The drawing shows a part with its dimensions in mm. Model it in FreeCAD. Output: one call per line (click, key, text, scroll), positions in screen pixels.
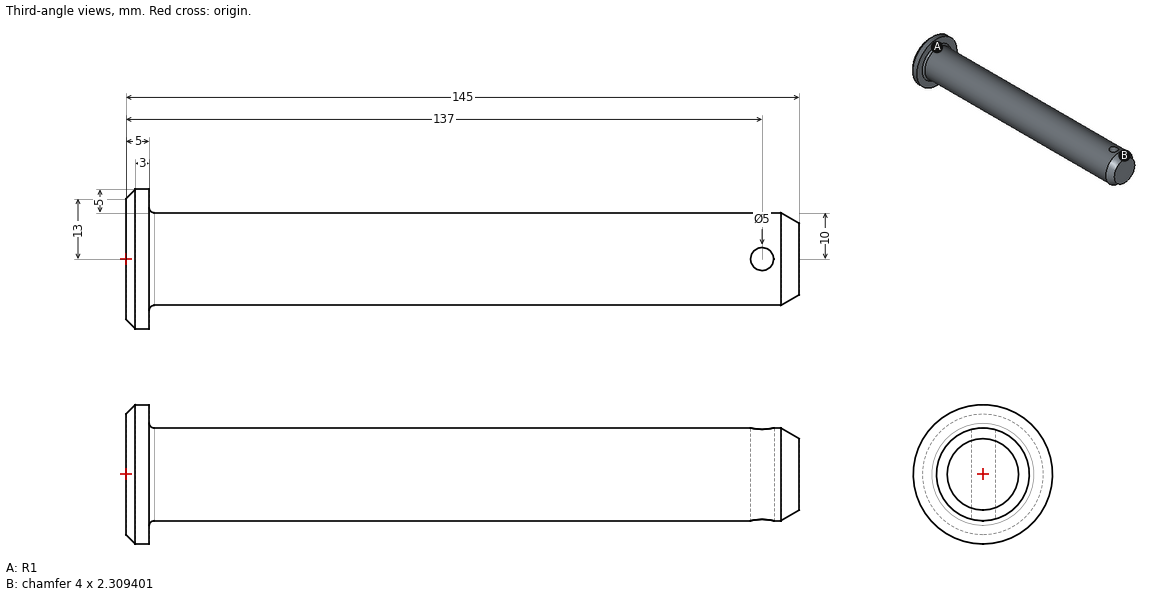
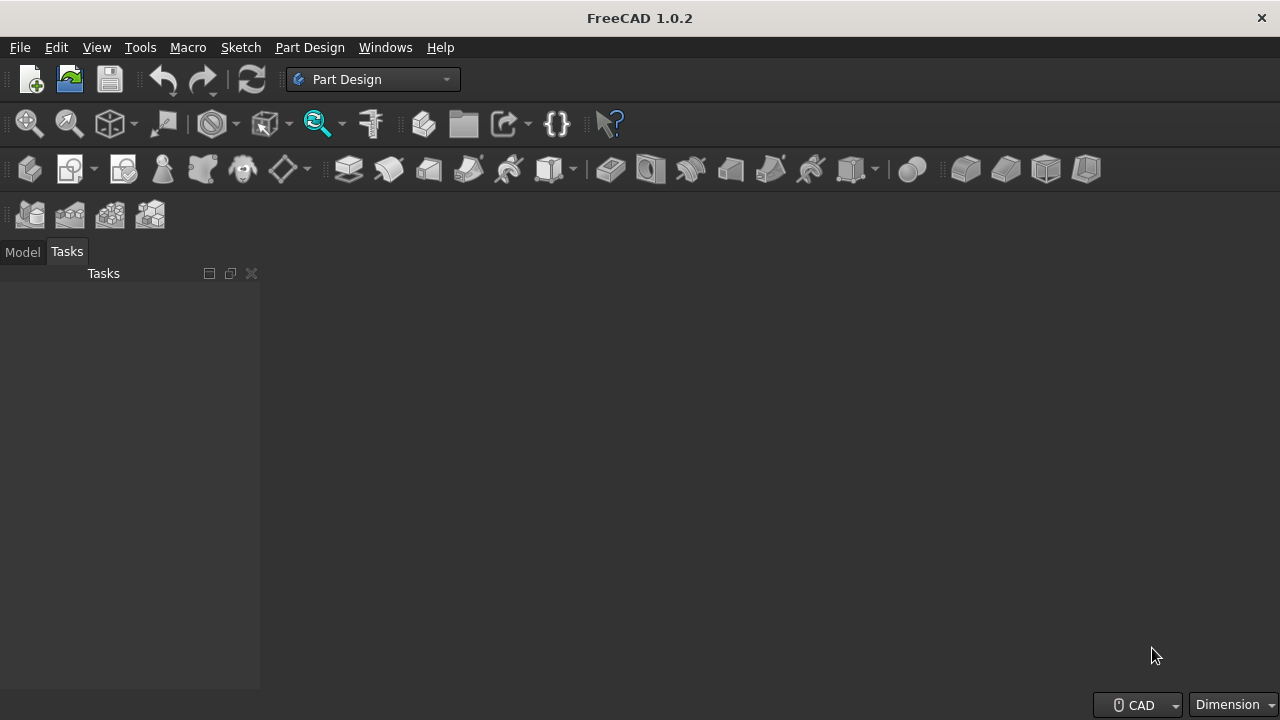
key(ctrl+n)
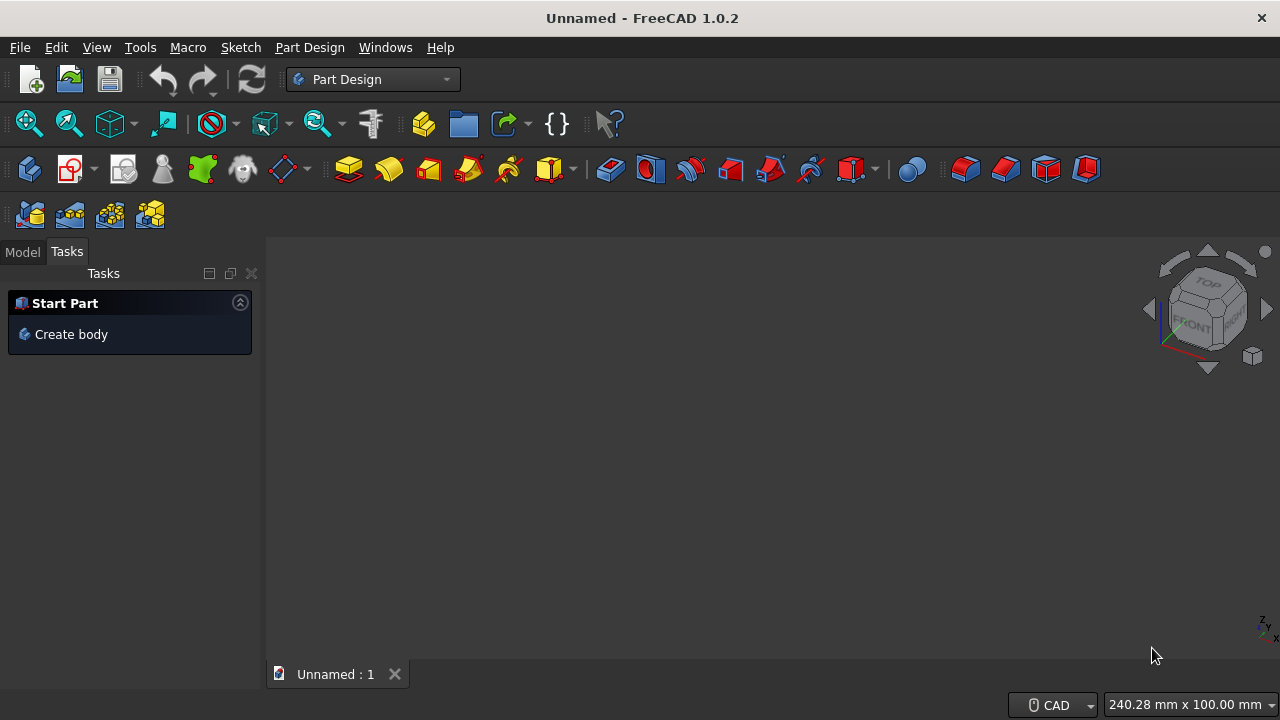
click(70, 170)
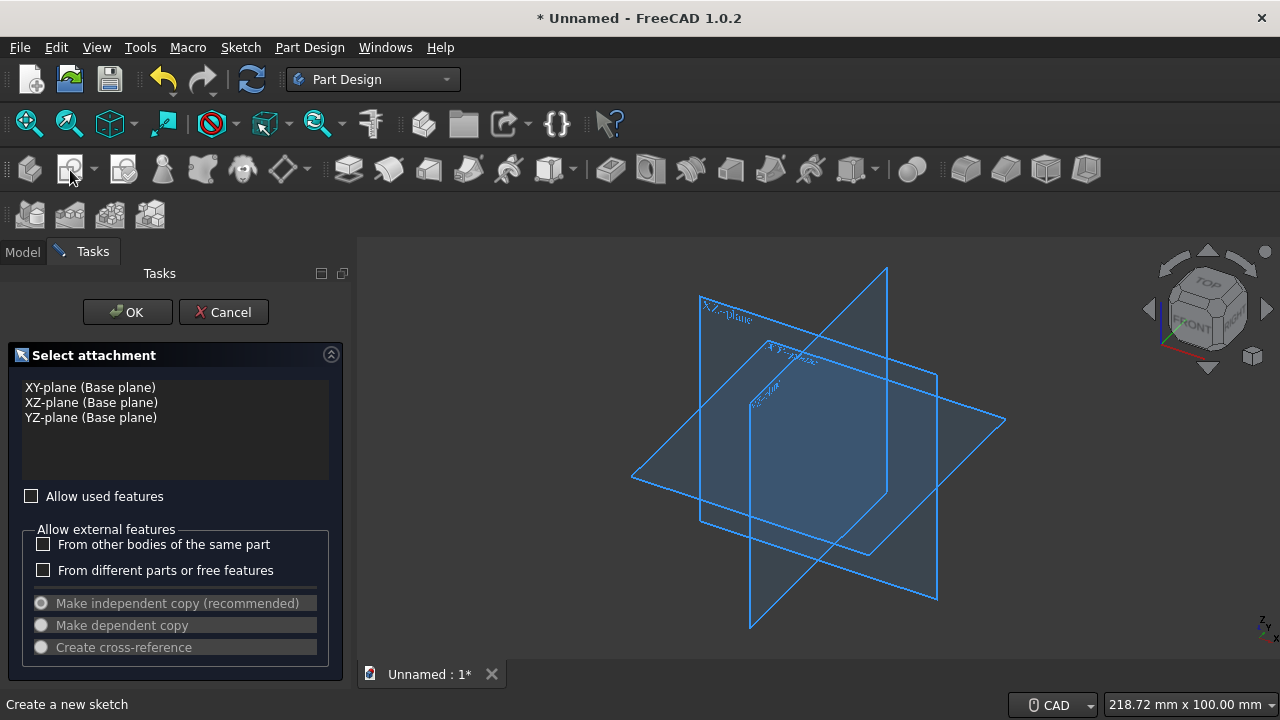
click(82, 388)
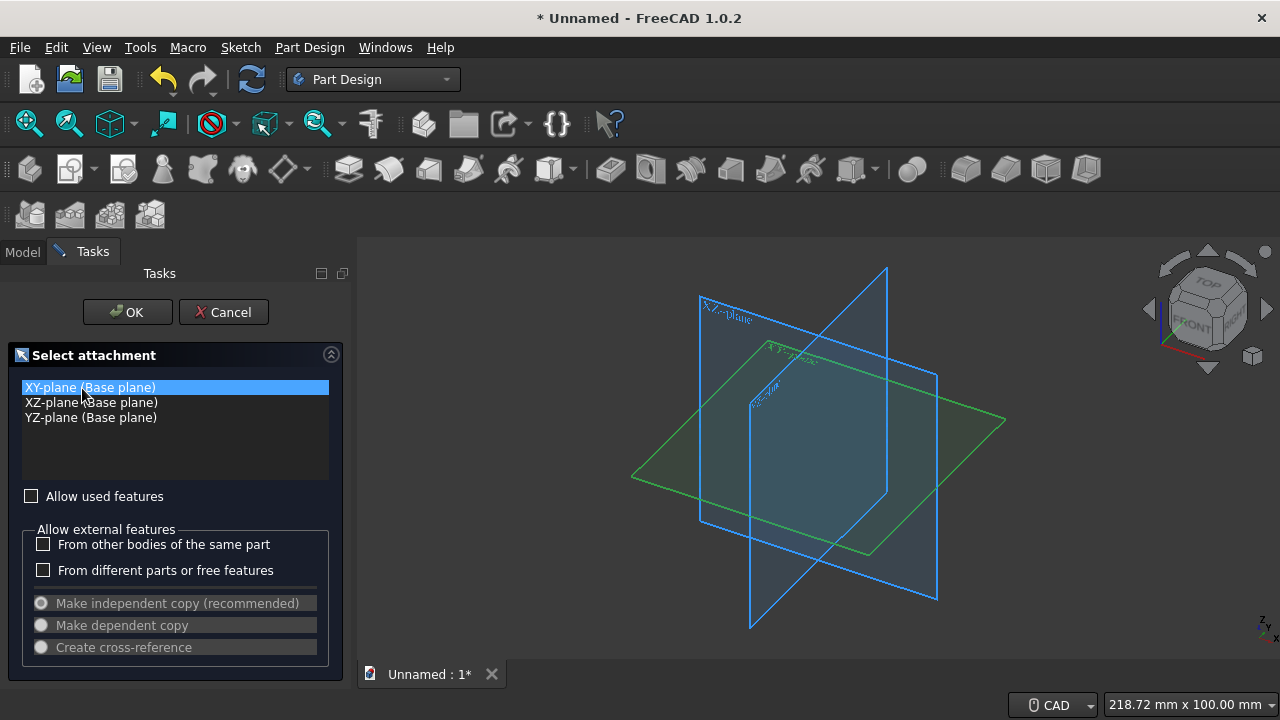
click(128, 312)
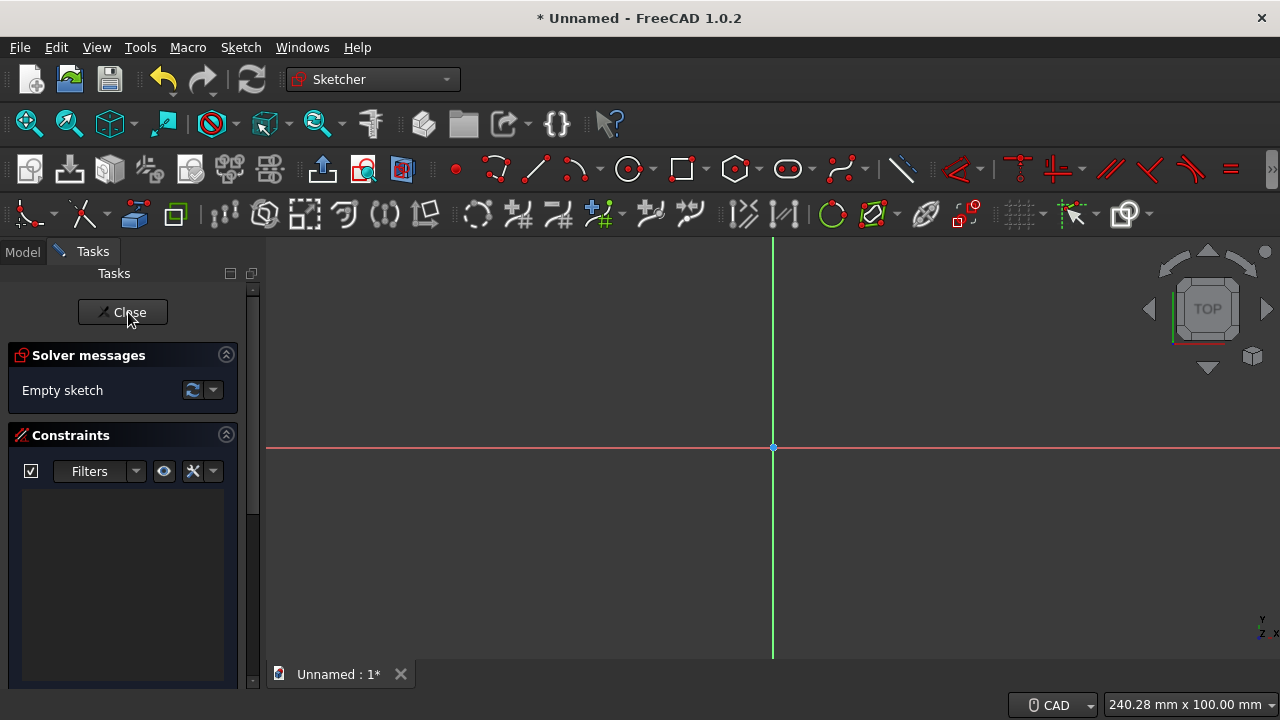
scroll(294, 512, down, 2)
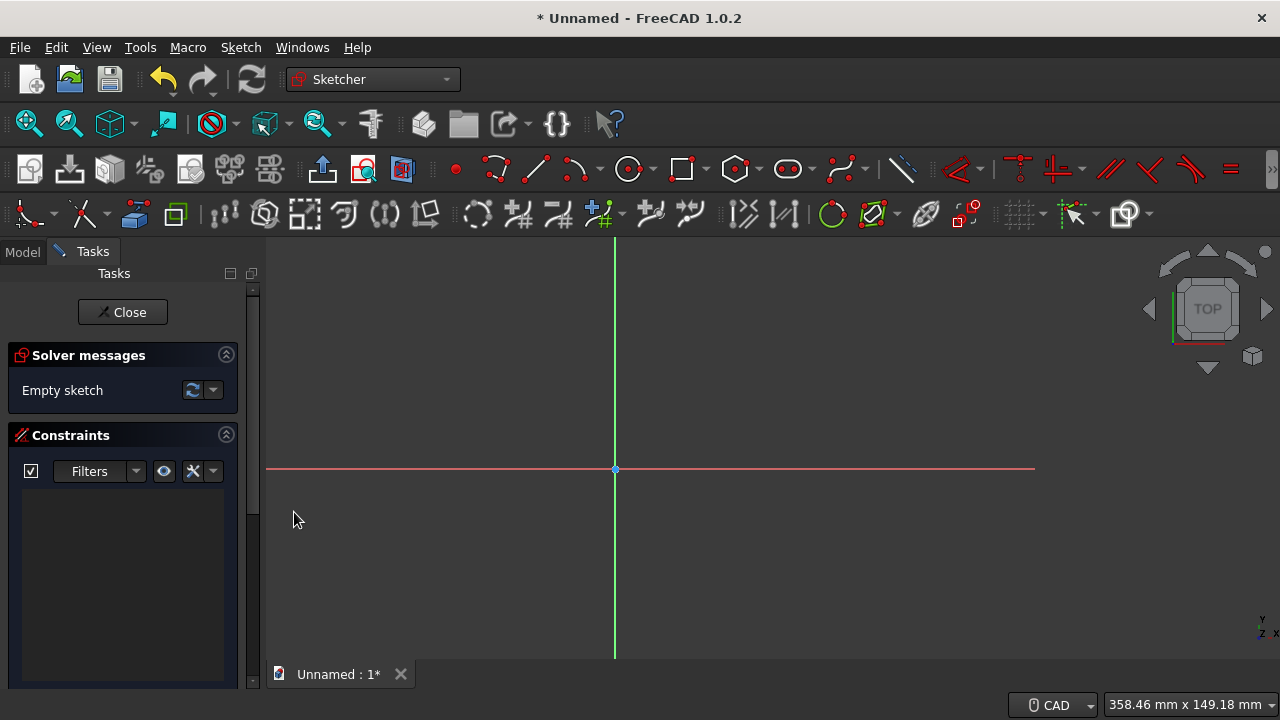
scroll(1055, 448, up, 2)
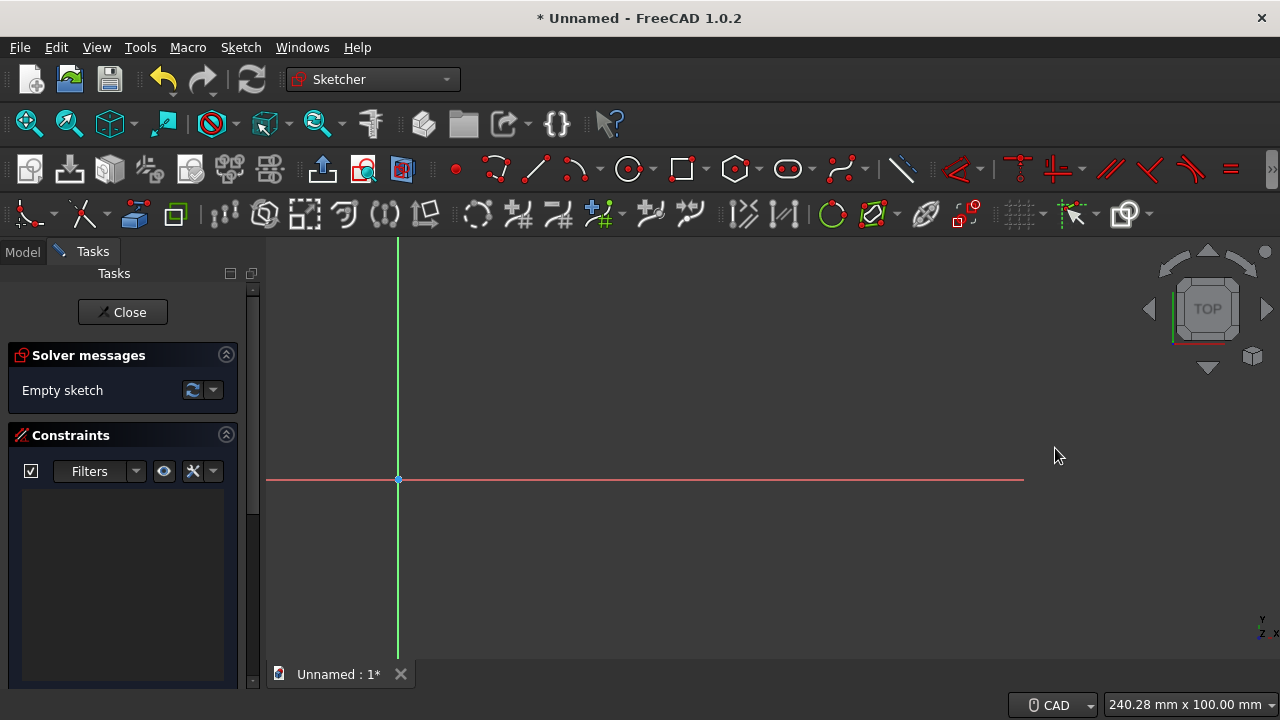
key(g)
key(m)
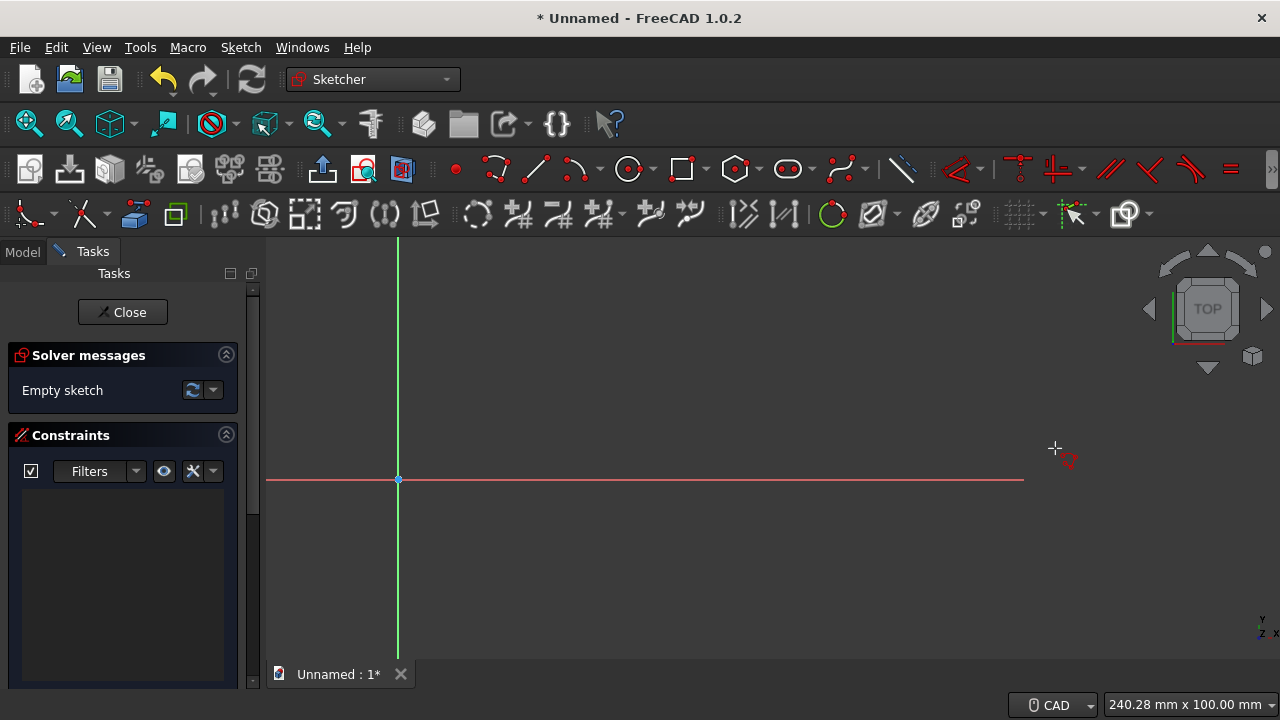
click(398, 480)
click(1010, 471)
click(1010, 437)
click(419, 437)
click(419, 416)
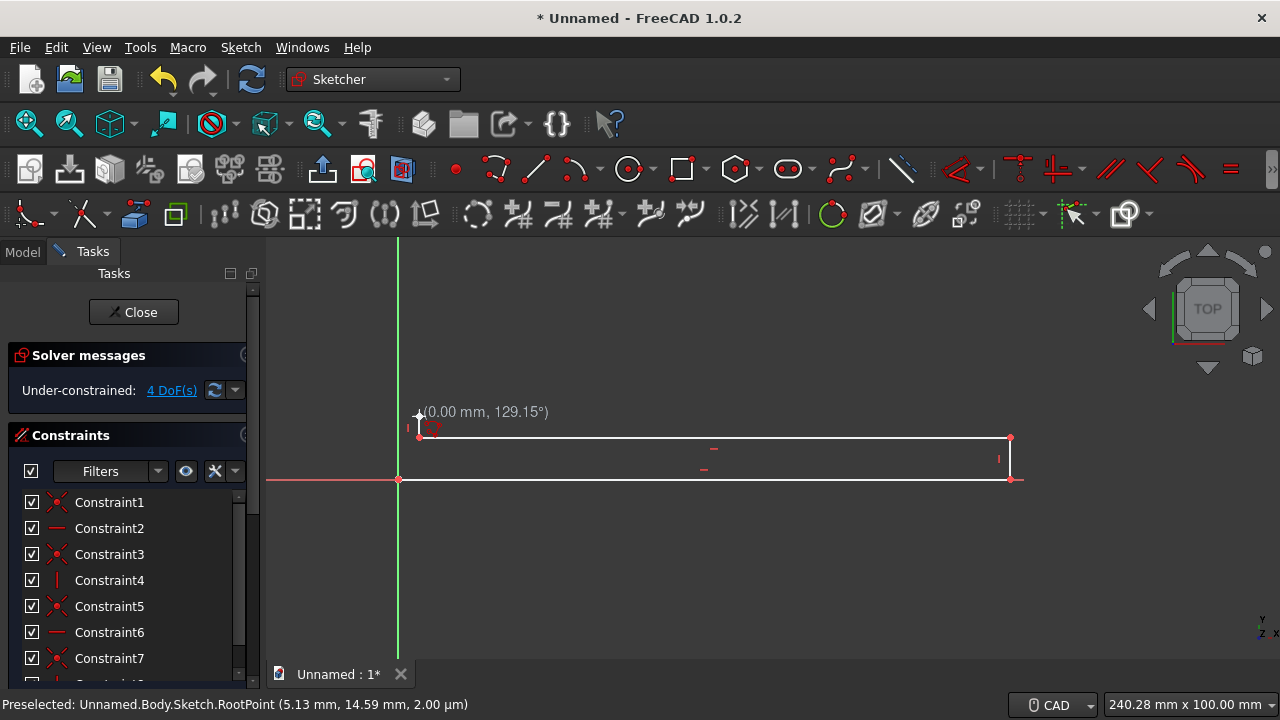
scroll(407, 416, up, 4)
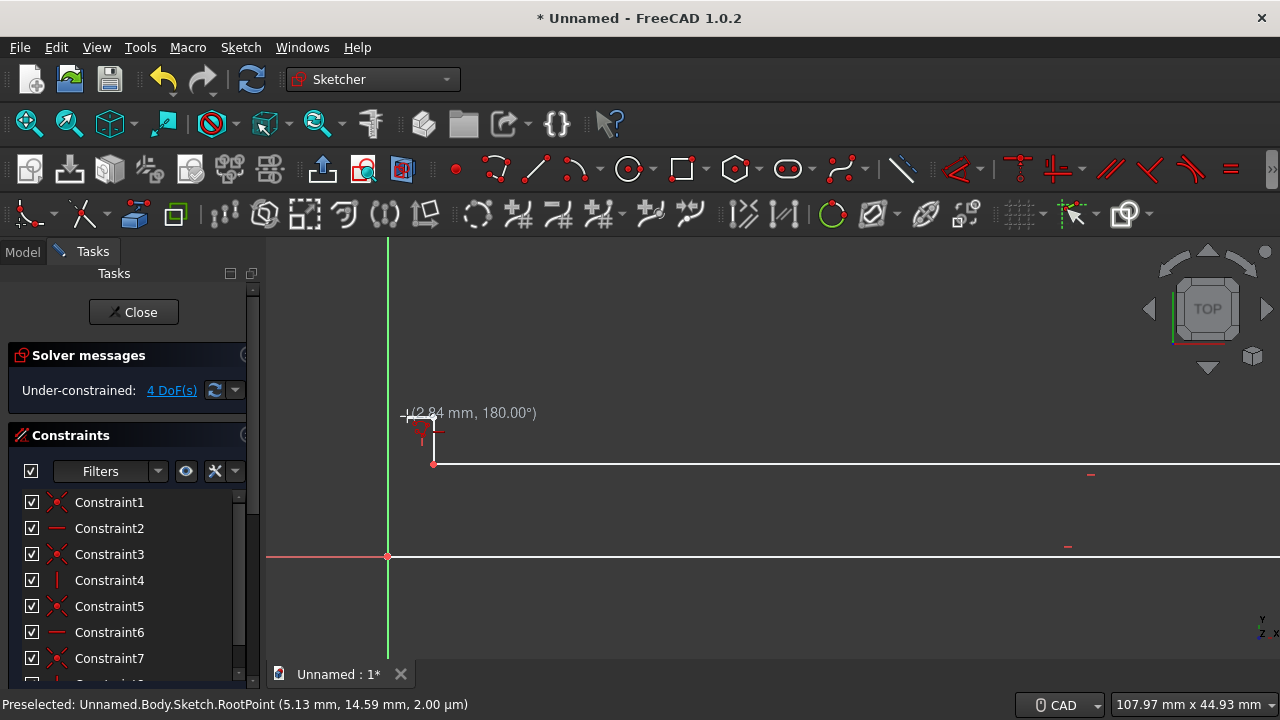
click(406, 415)
click(397, 435)
click(388, 557)
key(Escape)
key(Escape)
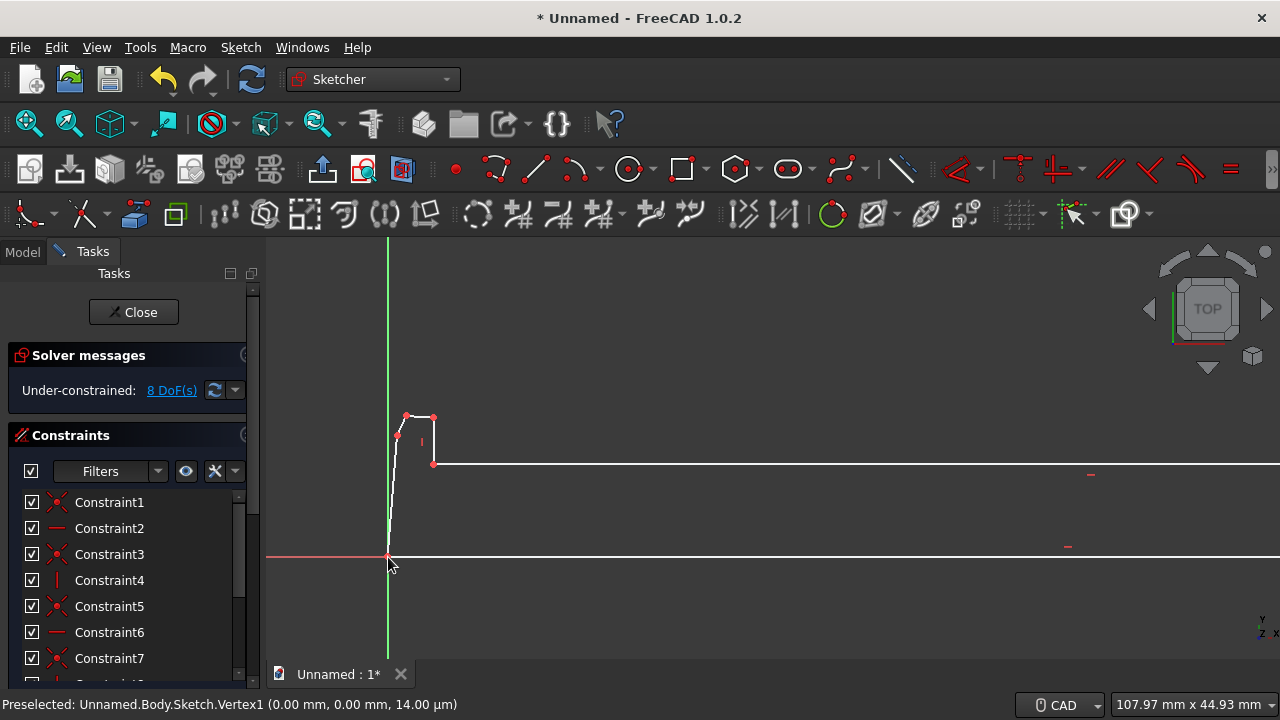
scroll(423, 417, up, 2)